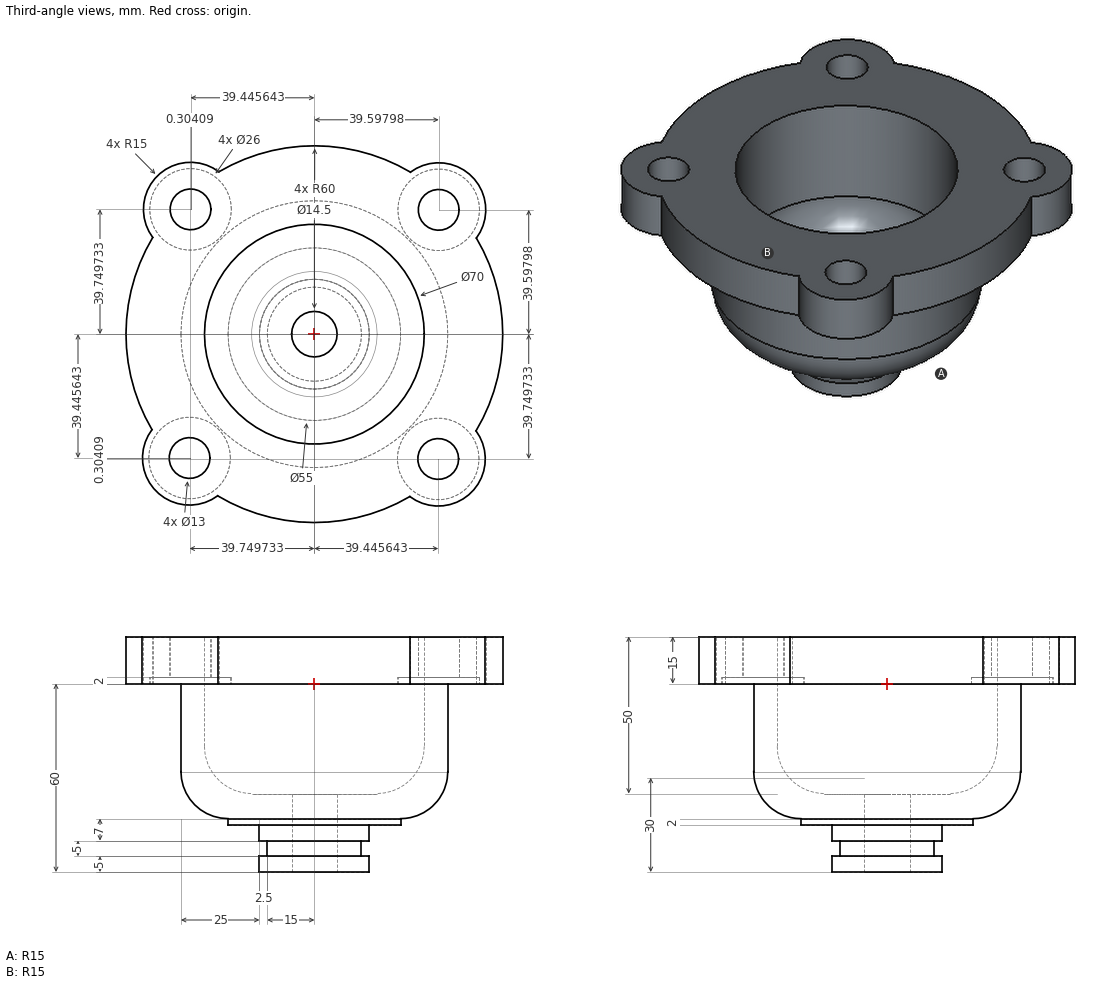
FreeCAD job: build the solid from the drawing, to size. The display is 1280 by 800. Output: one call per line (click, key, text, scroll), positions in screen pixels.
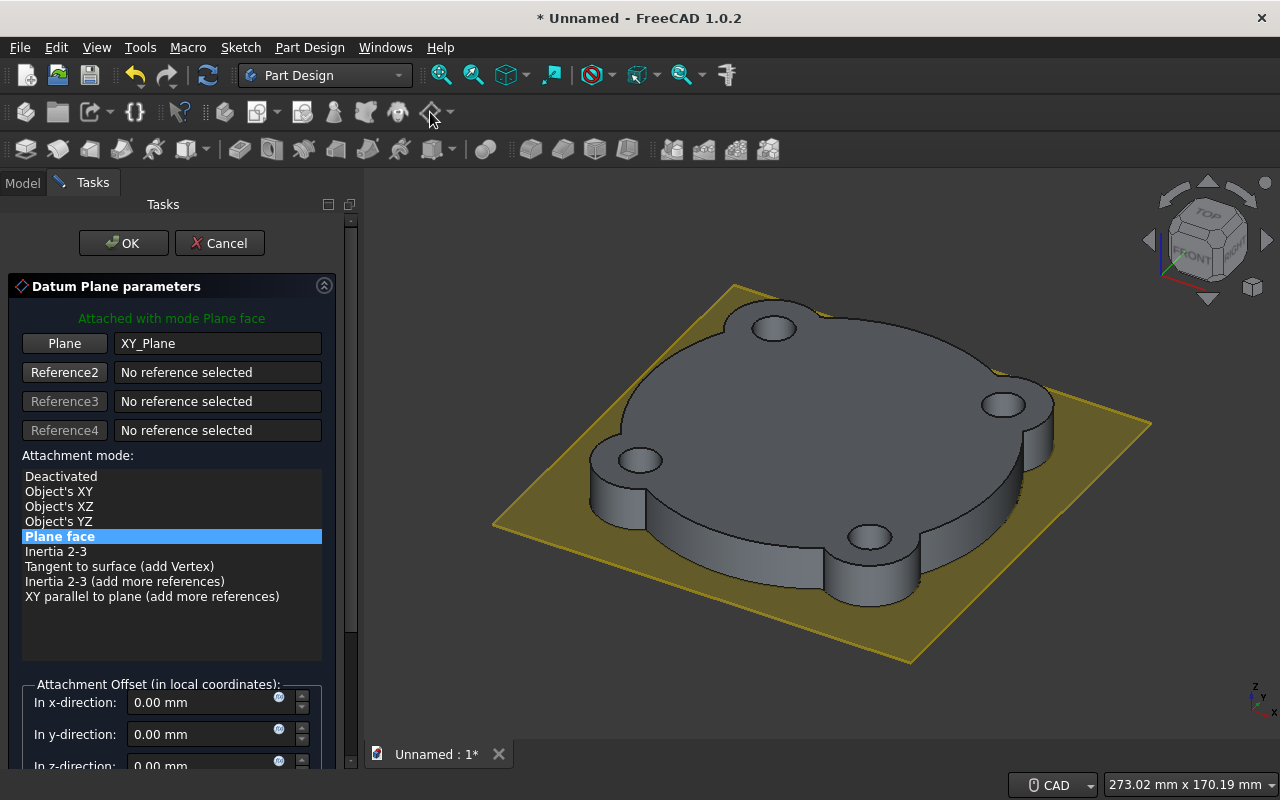
scroll(351, 491, down, 2)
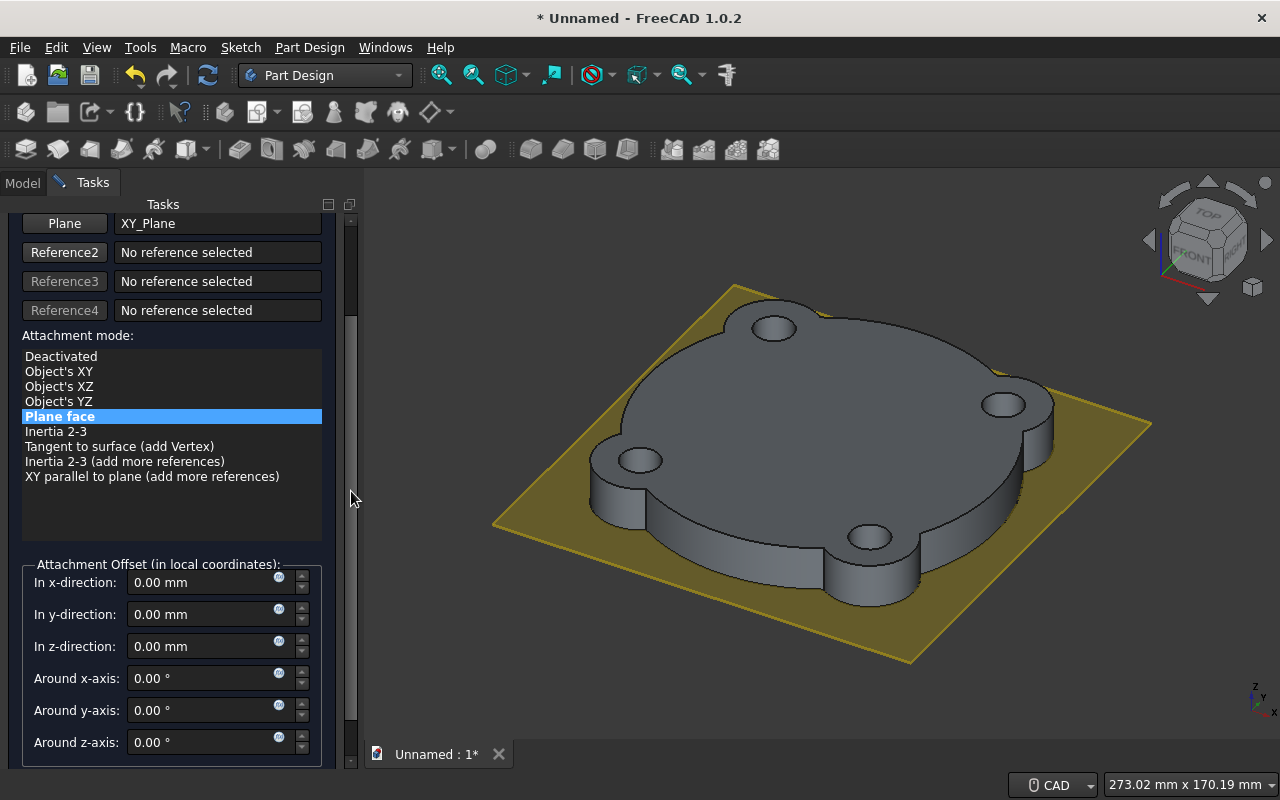
triple_click(210, 646)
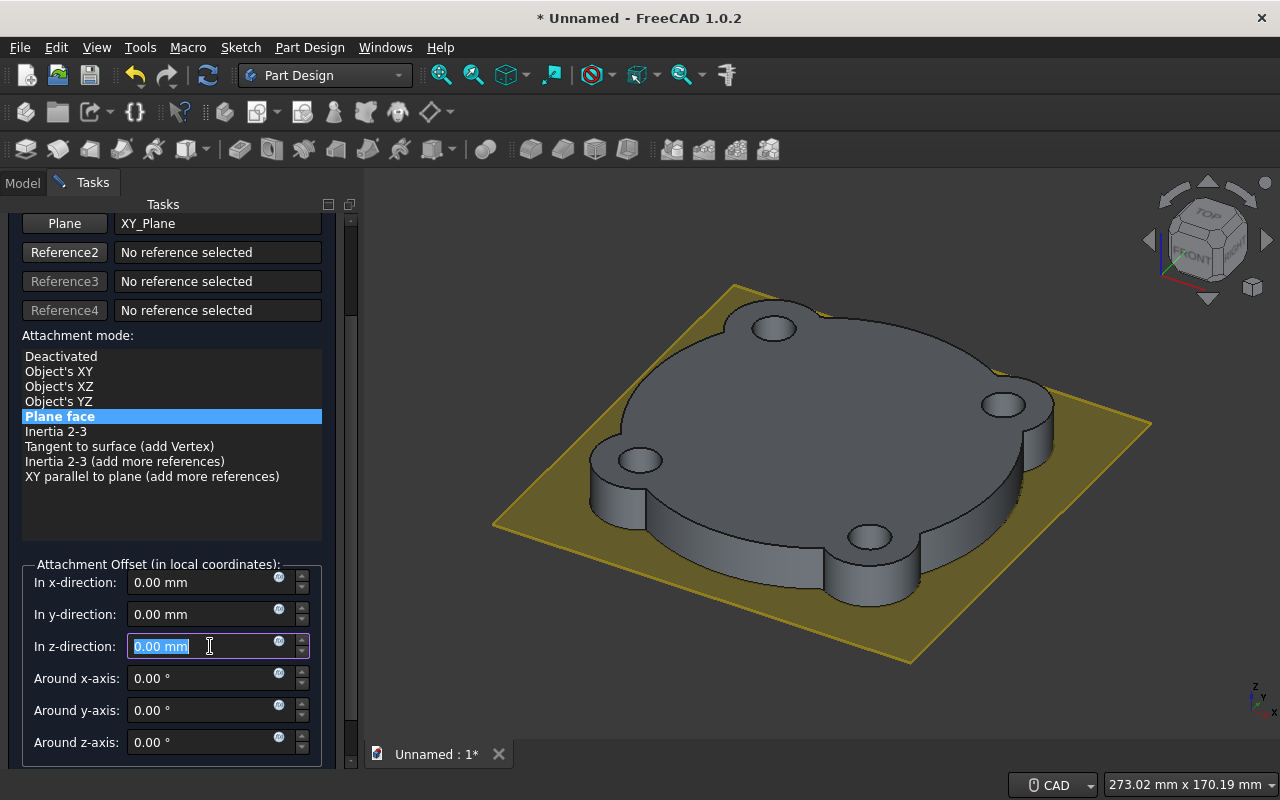
text(2)
key(Tab)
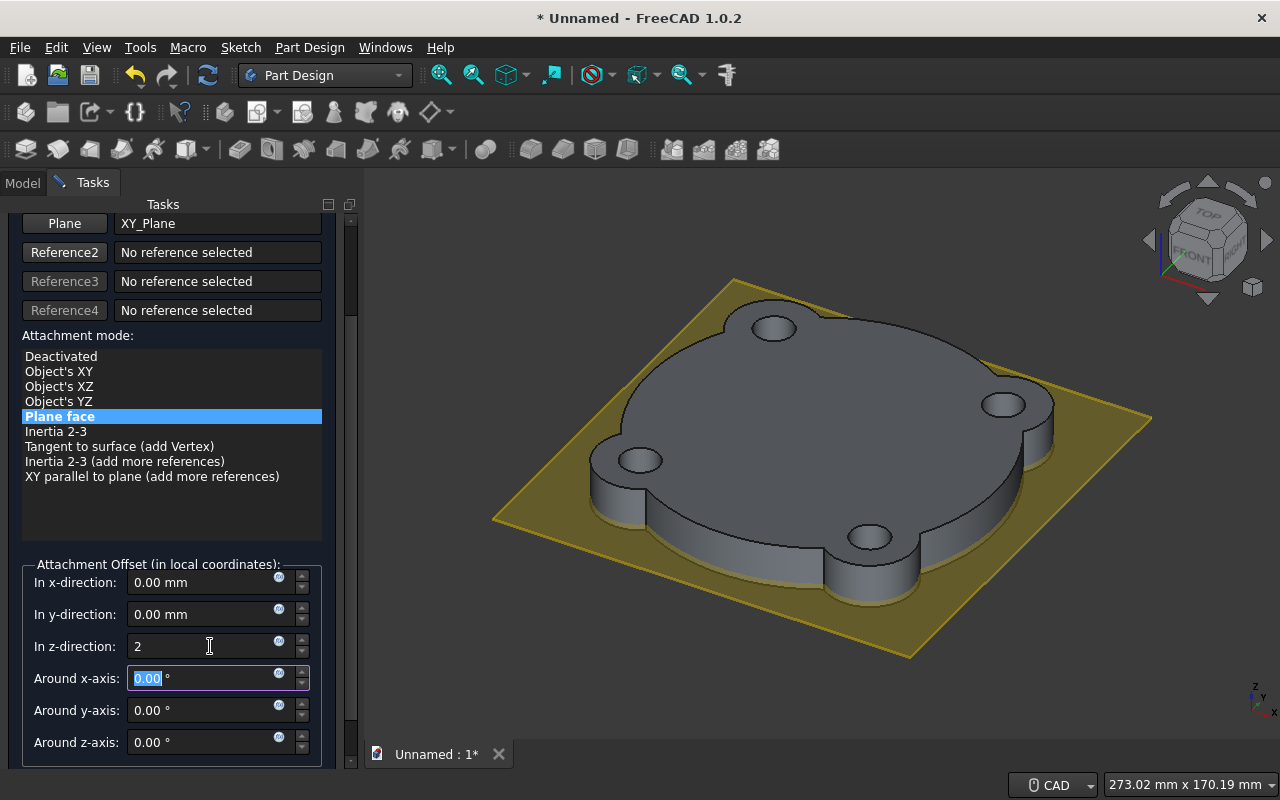
scroll(351, 491, up, 3)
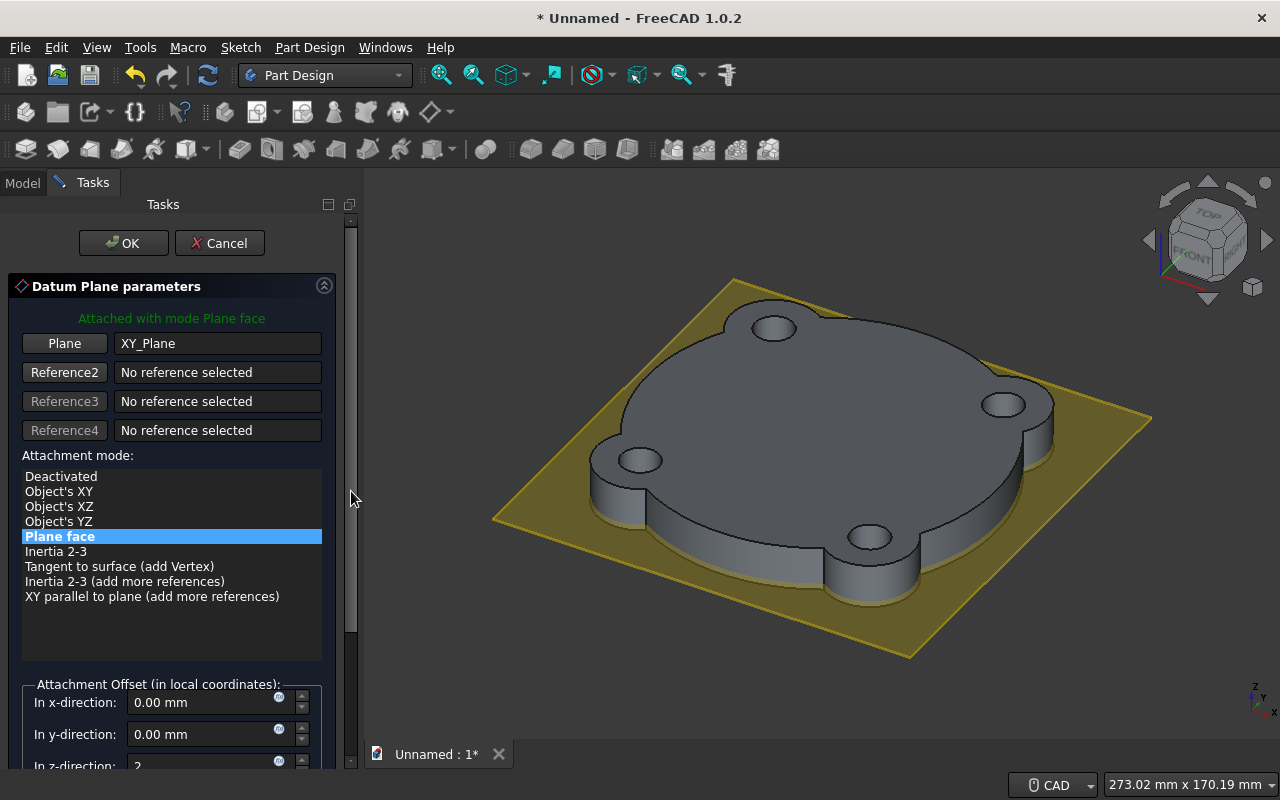
click(124, 243)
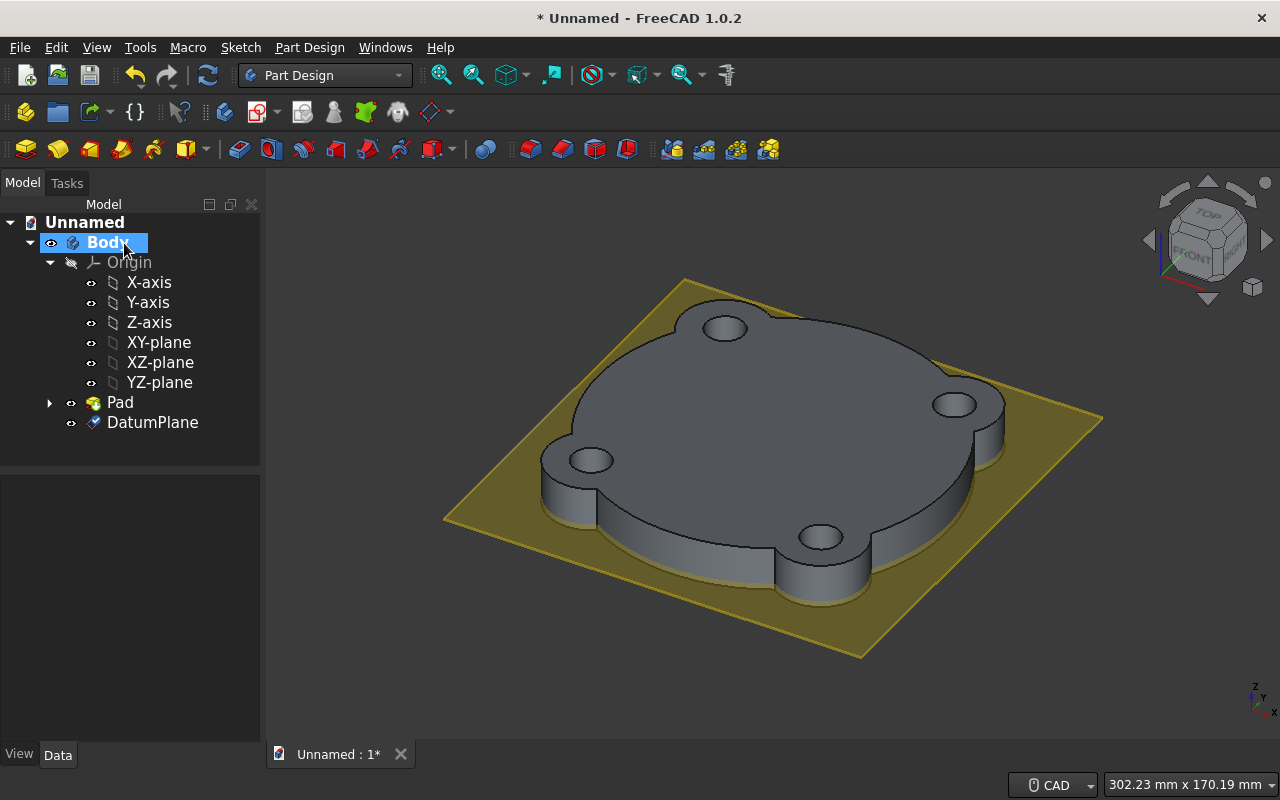
click(116, 423)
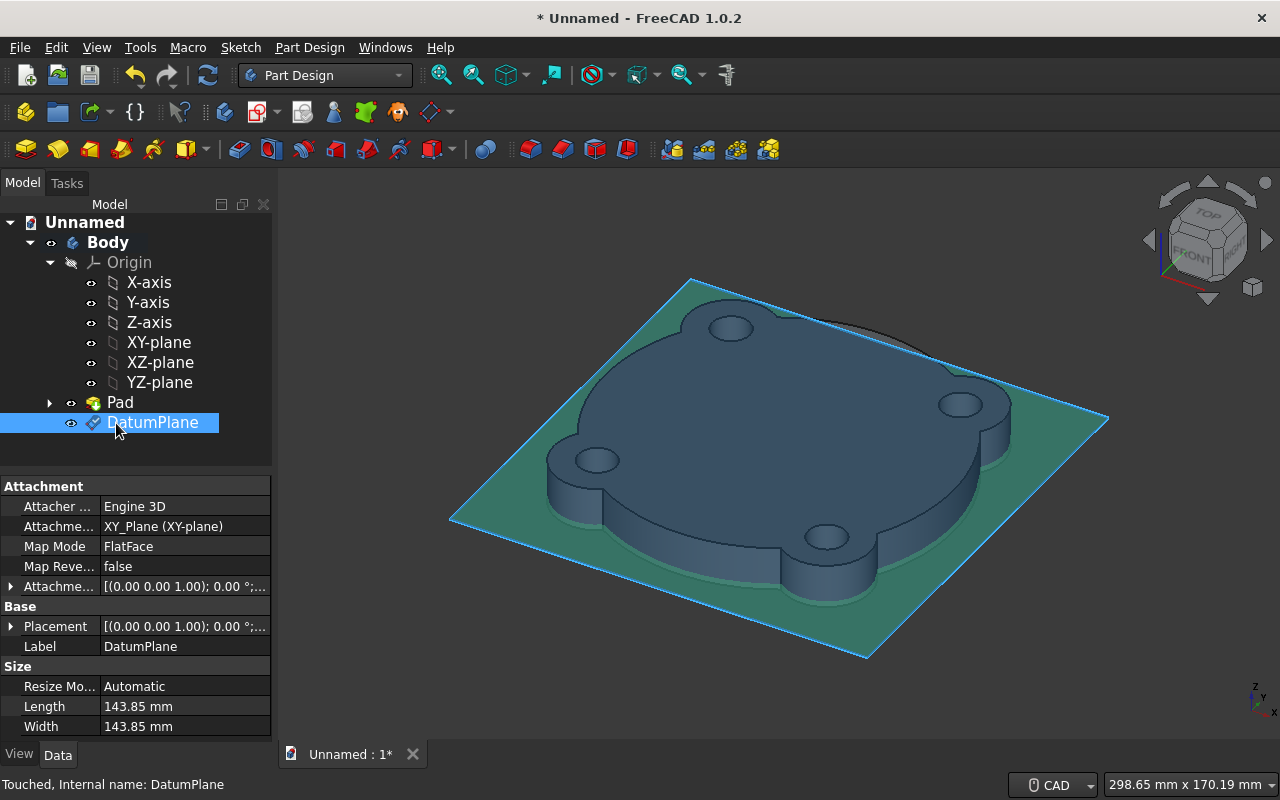
click(258, 112)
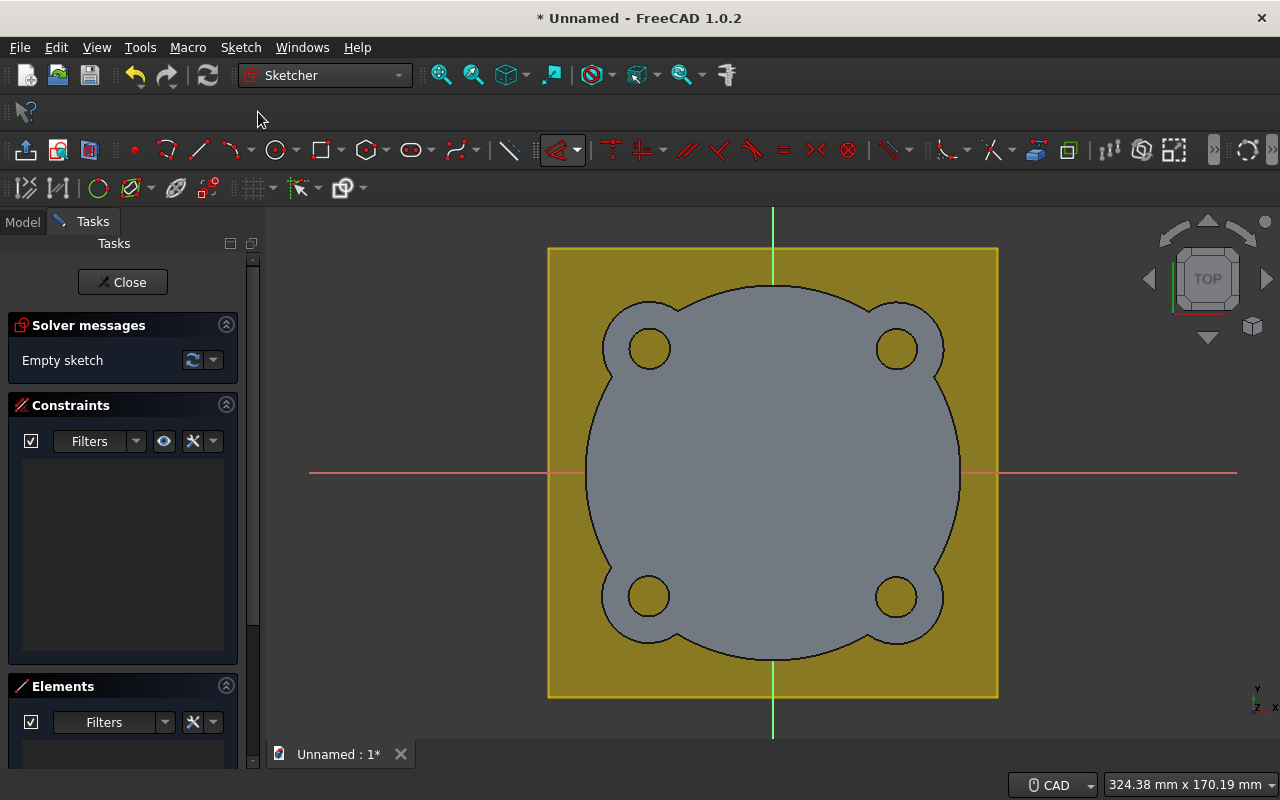
click(90, 150)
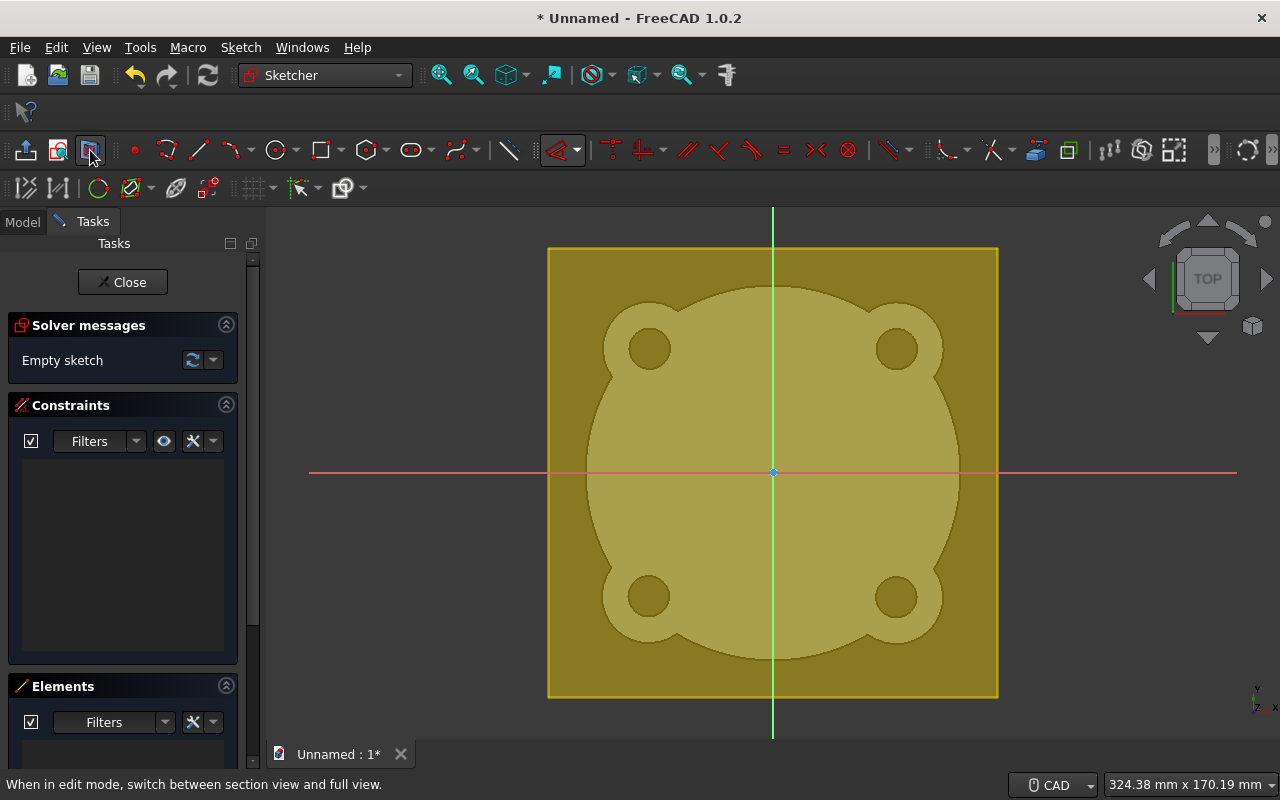
key(g)
key(c)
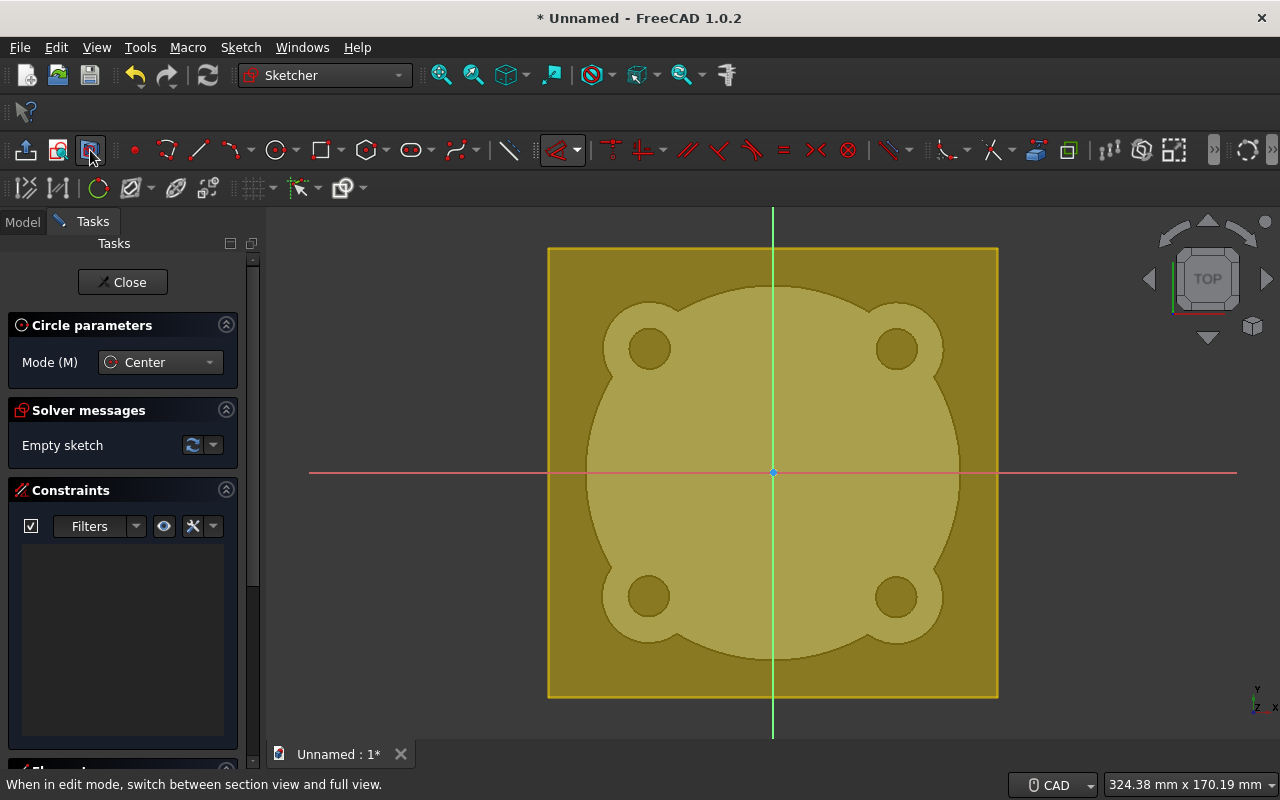
click(650, 349)
move(678, 320)